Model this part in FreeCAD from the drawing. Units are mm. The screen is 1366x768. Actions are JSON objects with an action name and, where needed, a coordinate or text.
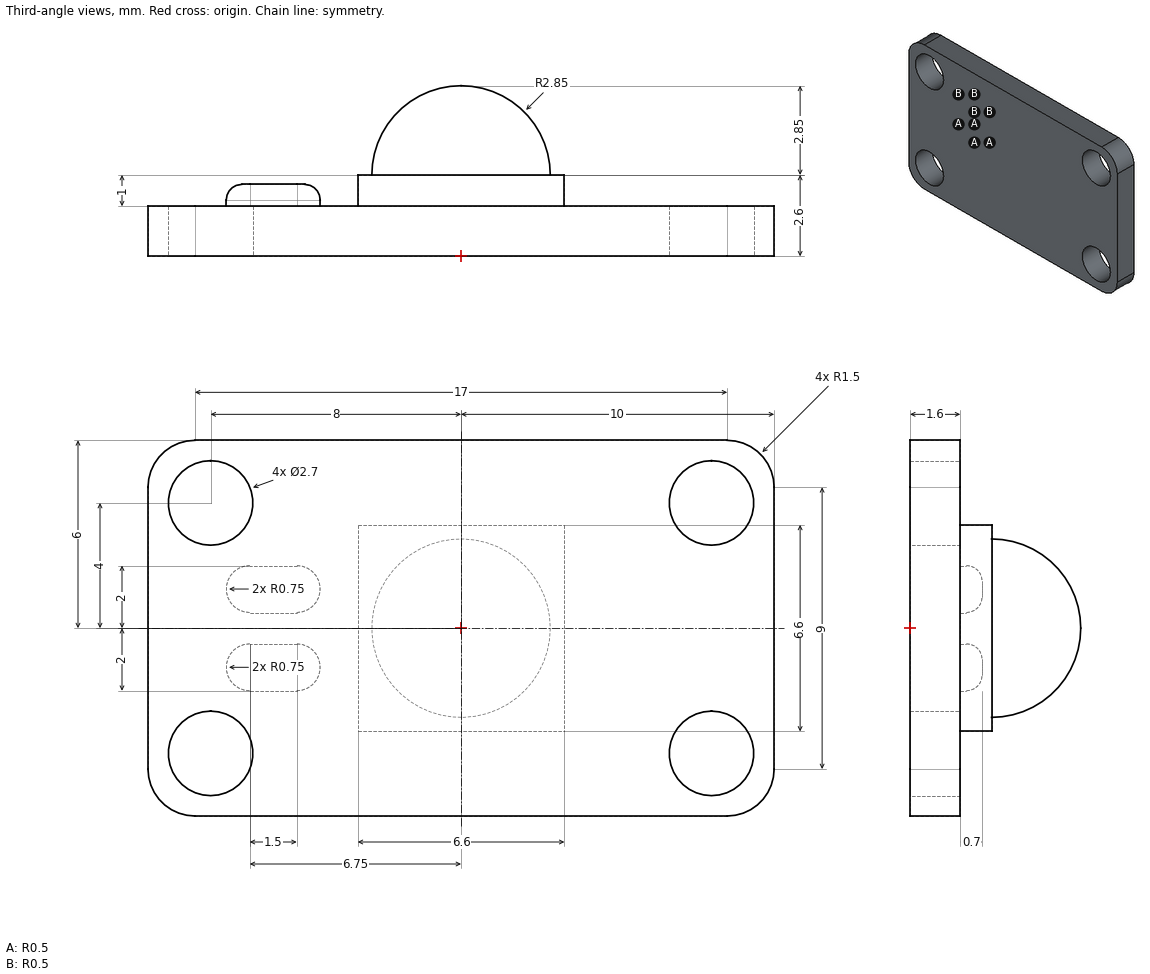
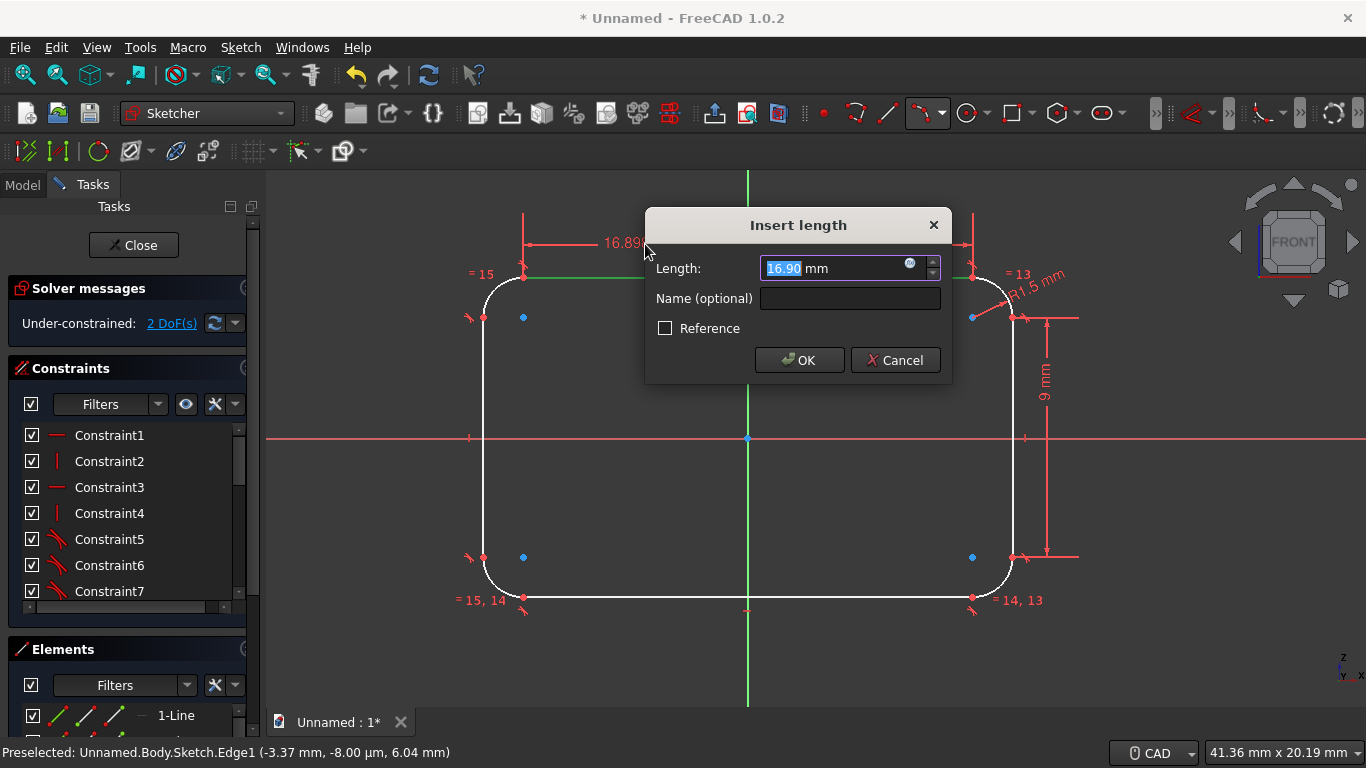
{"action": "type", "text": "17"}
{"action": "key", "text": "Return"}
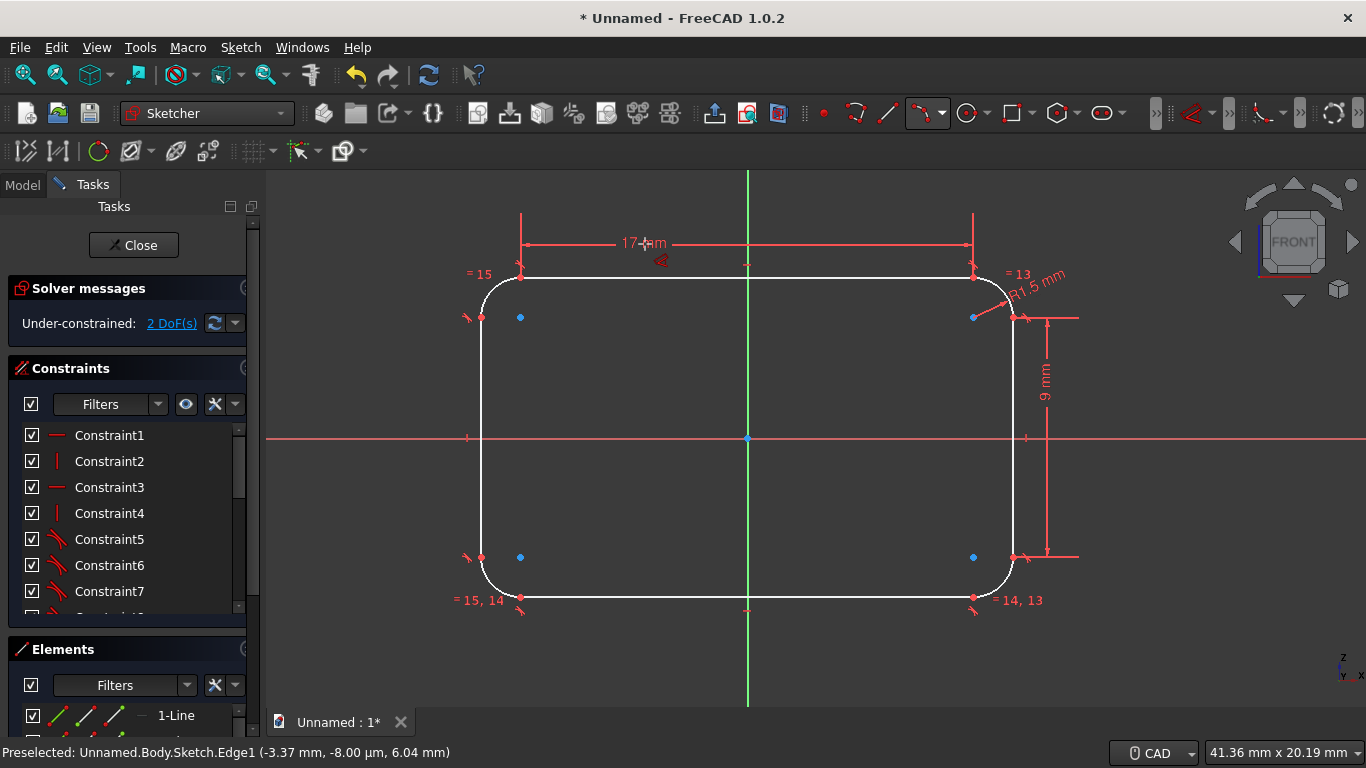
{"action": "left_click", "coordinate": [521, 278]}
{"action": "left_click", "coordinate": [782, 358]}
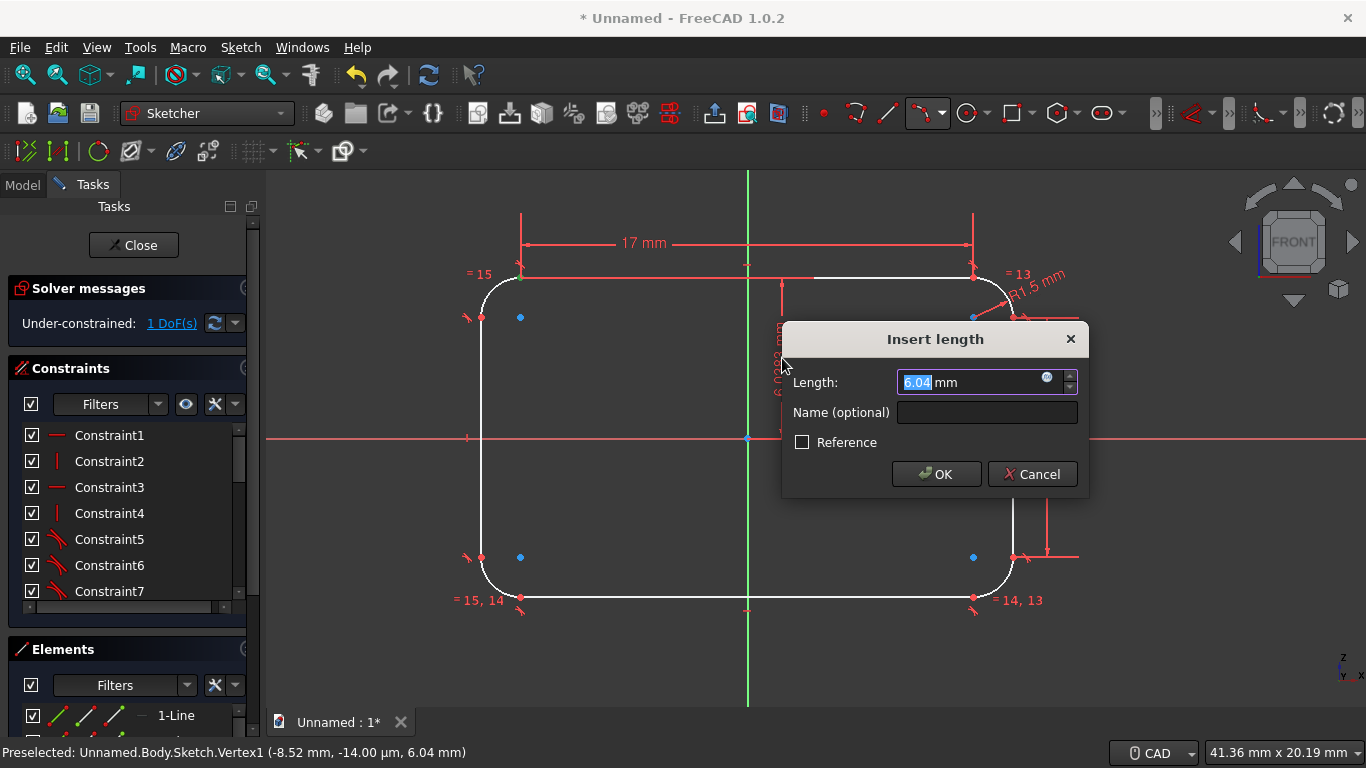
{"action": "type", "text": "6"}
{"action": "key", "text": "Return"}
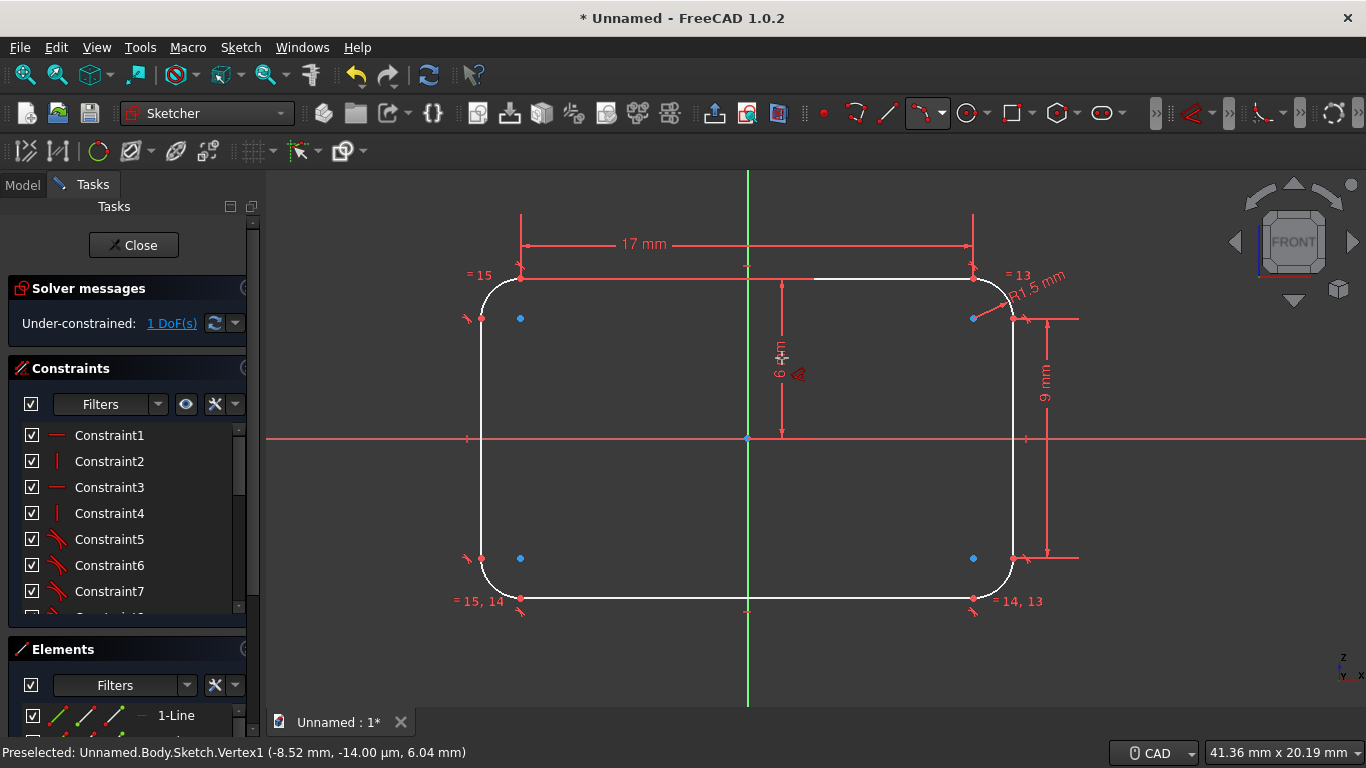
{"action": "left_click", "coordinate": [1013, 319]}
{"action": "left_click", "coordinate": [880, 473]}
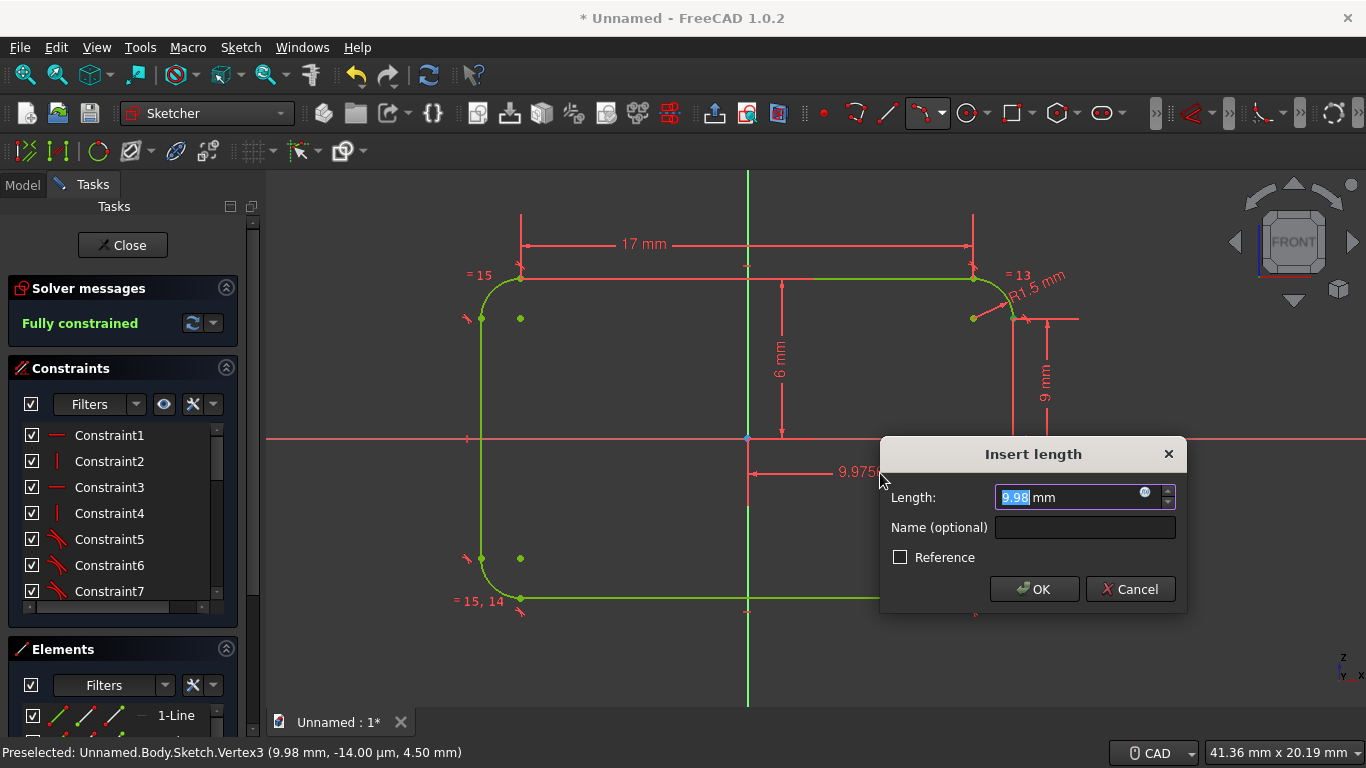
{"action": "type", "text": "10"}
{"action": "key", "text": "Return"}
{"action": "key", "text": "Escape"}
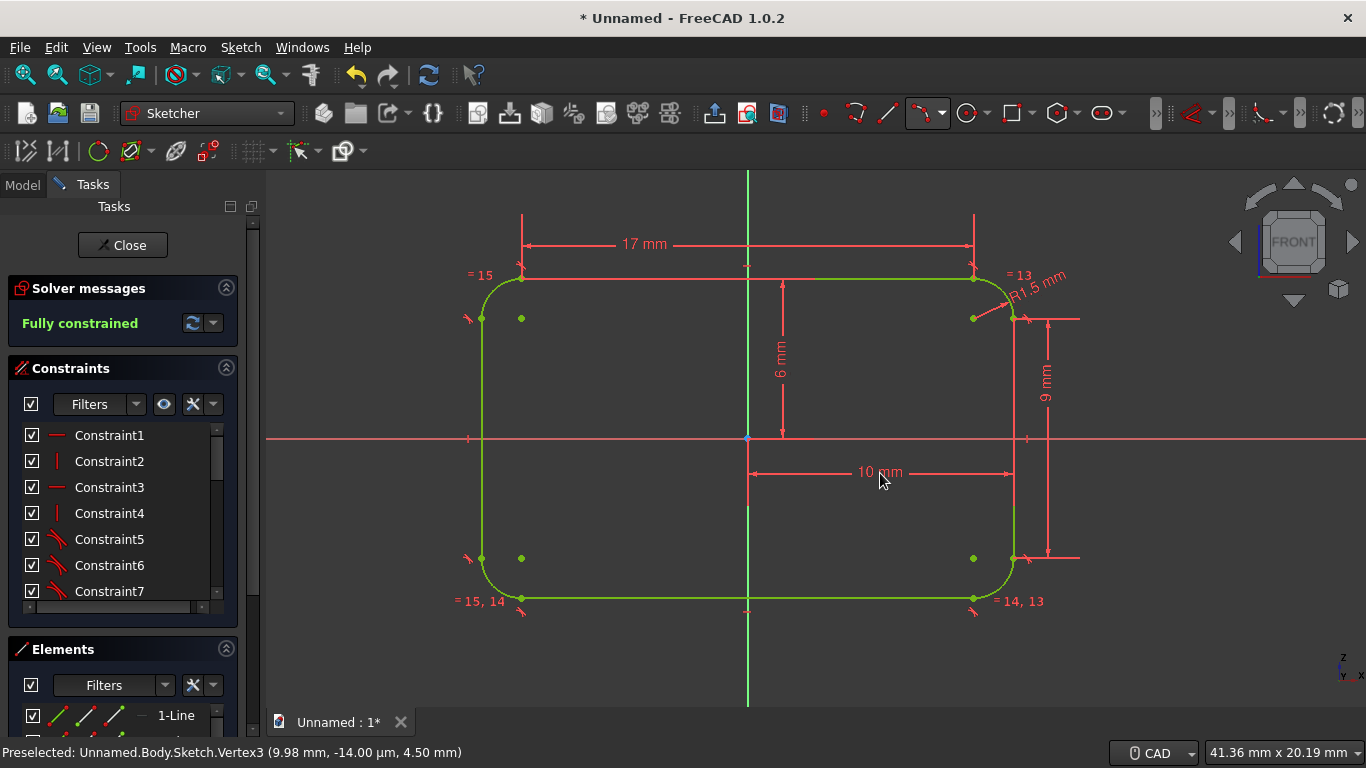
{"action": "left_click", "coordinate": [123, 245]}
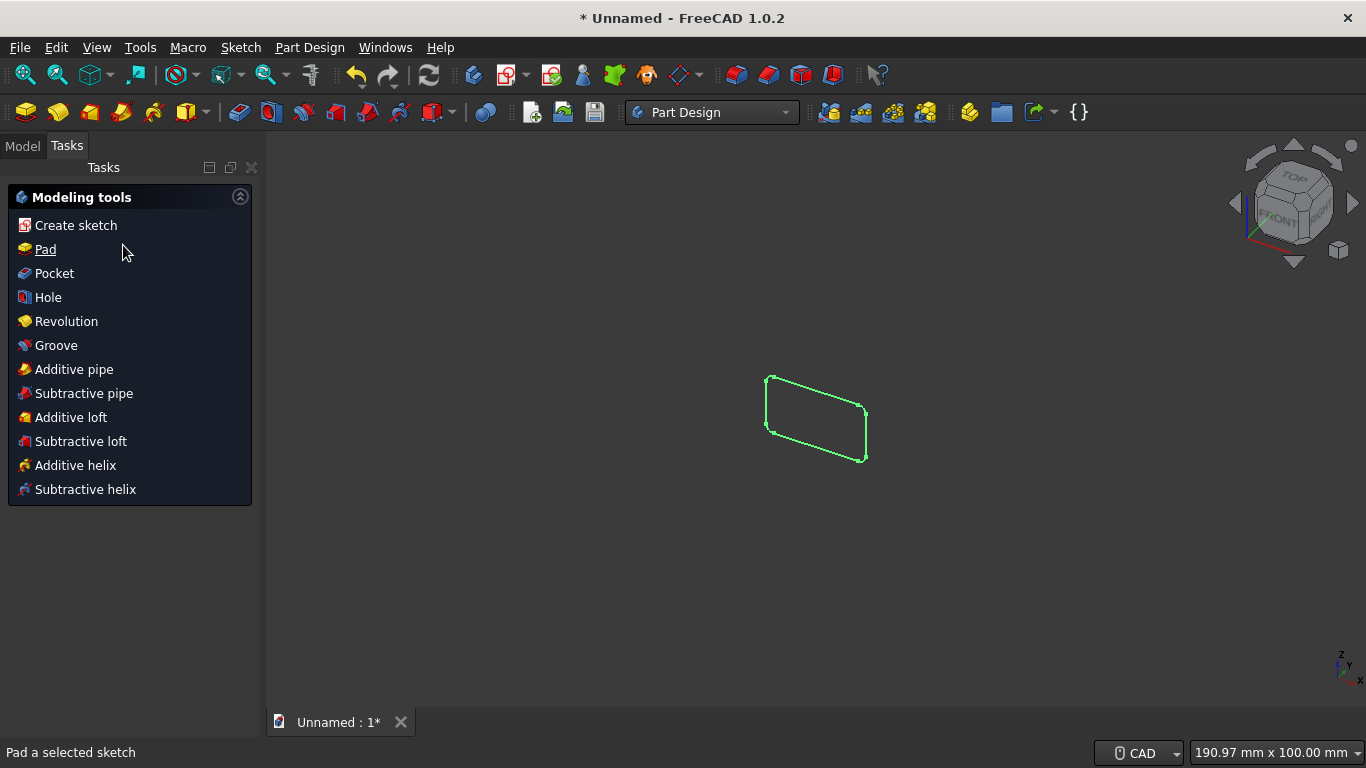
{"action": "left_click", "coordinate": [26, 112]}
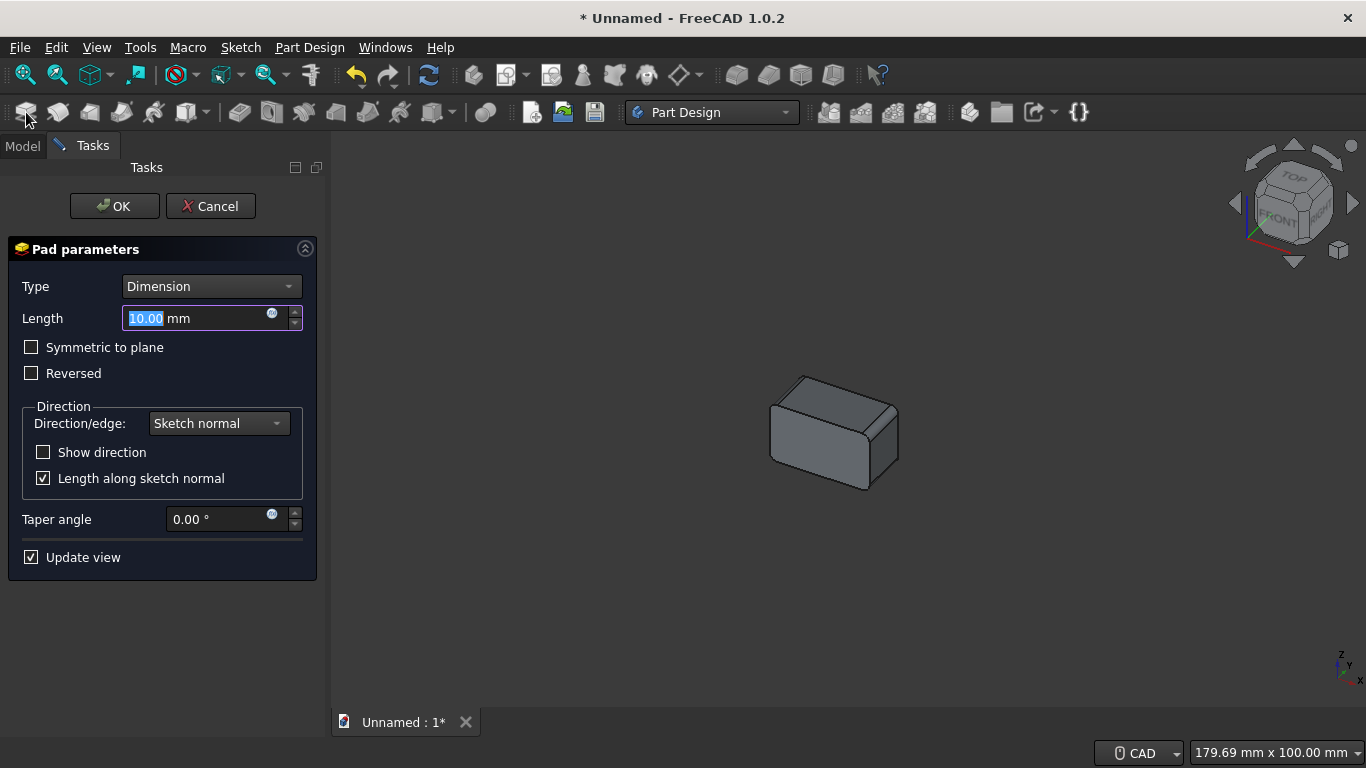
{"action": "type", "text": "1.6"}
{"action": "key", "text": "Tab"}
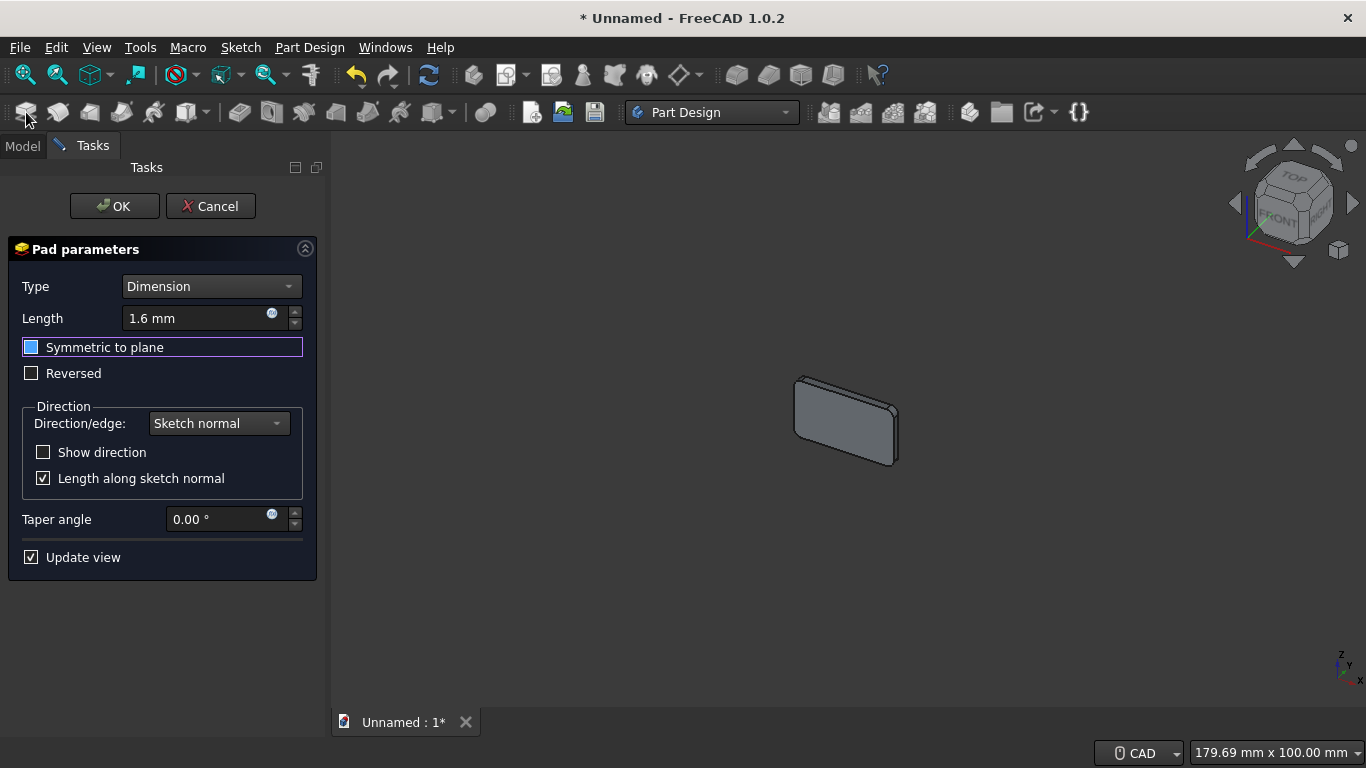
{"action": "left_click", "coordinate": [30, 373]}